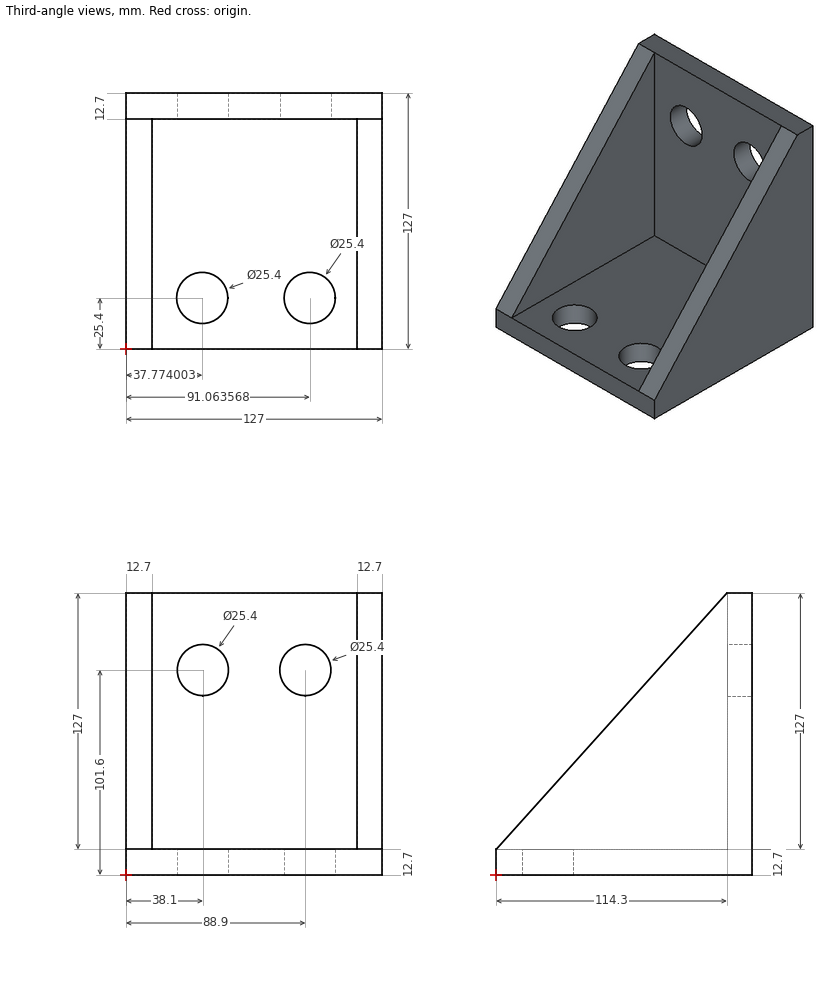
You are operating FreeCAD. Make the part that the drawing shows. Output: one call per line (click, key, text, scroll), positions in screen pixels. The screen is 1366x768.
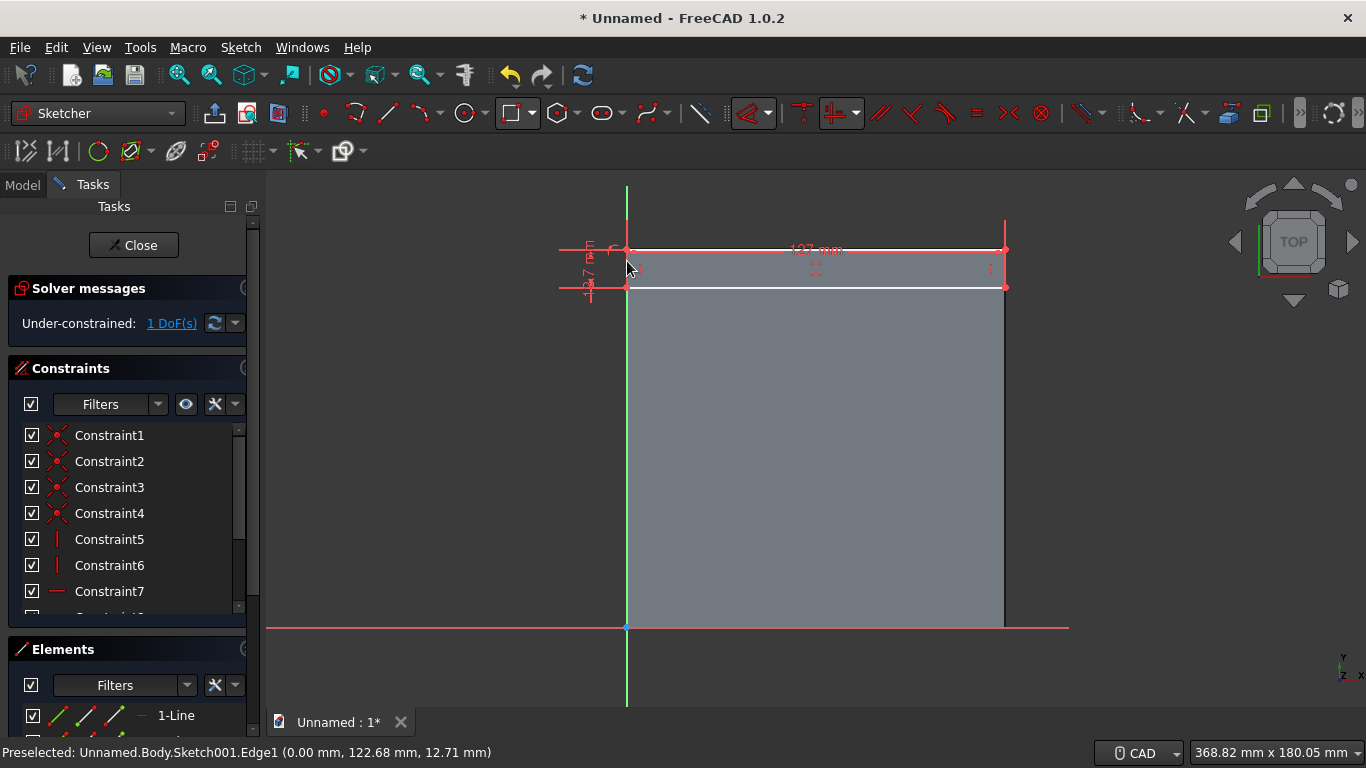
click(627, 250)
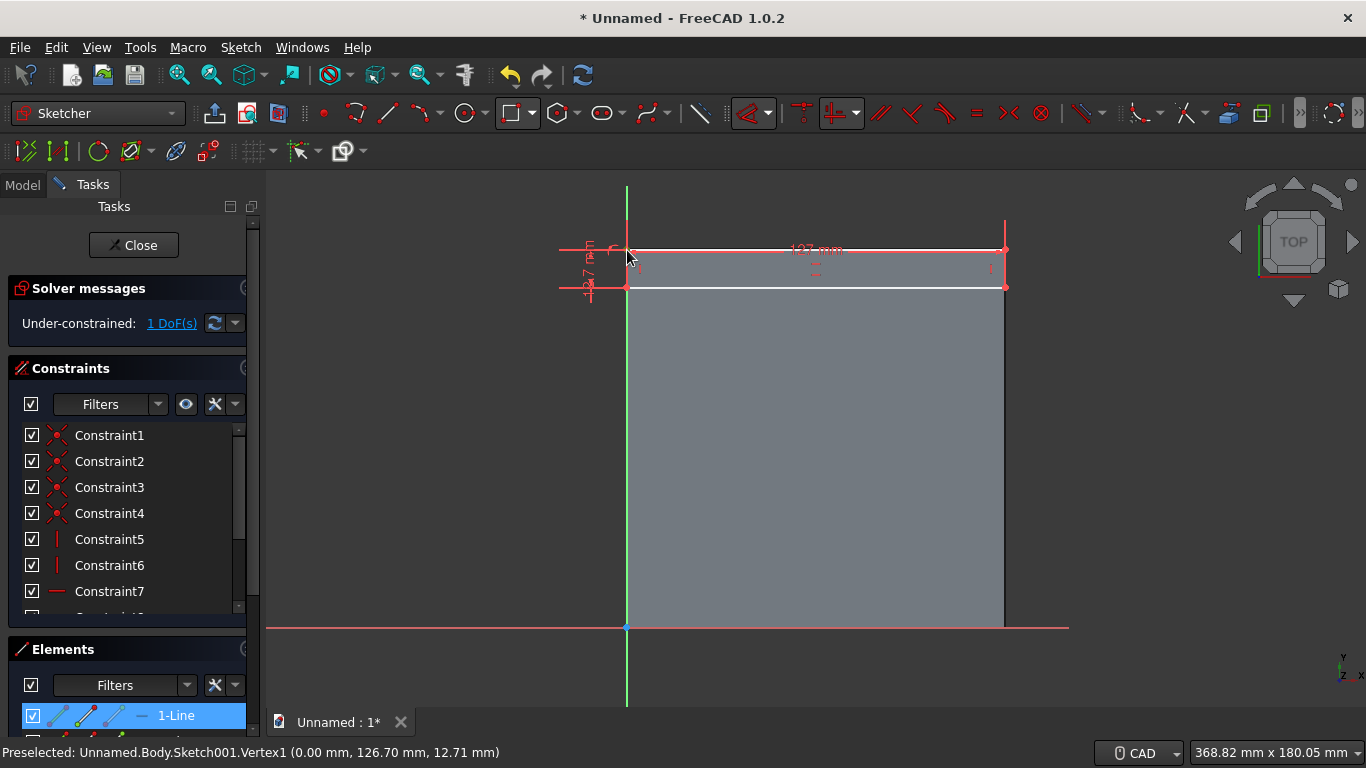
key(i)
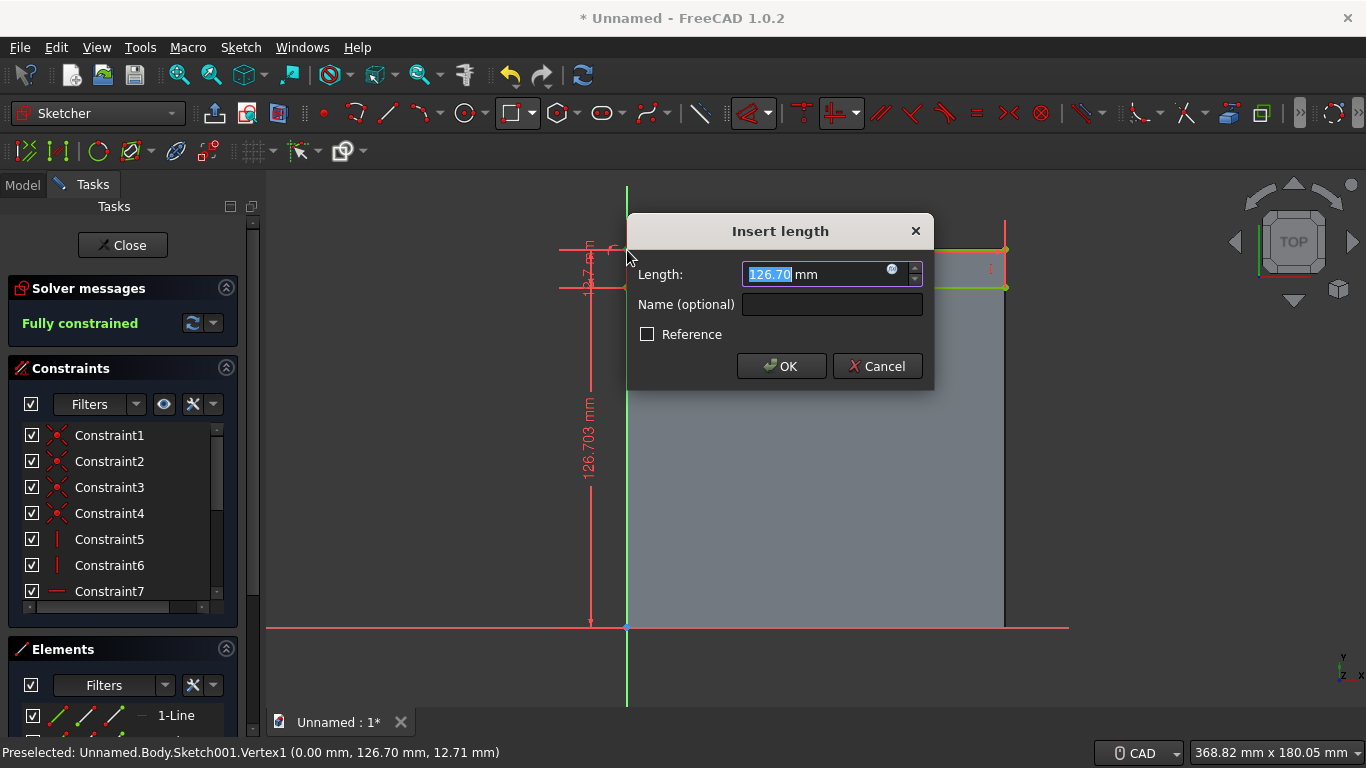
text(127)
key(Return)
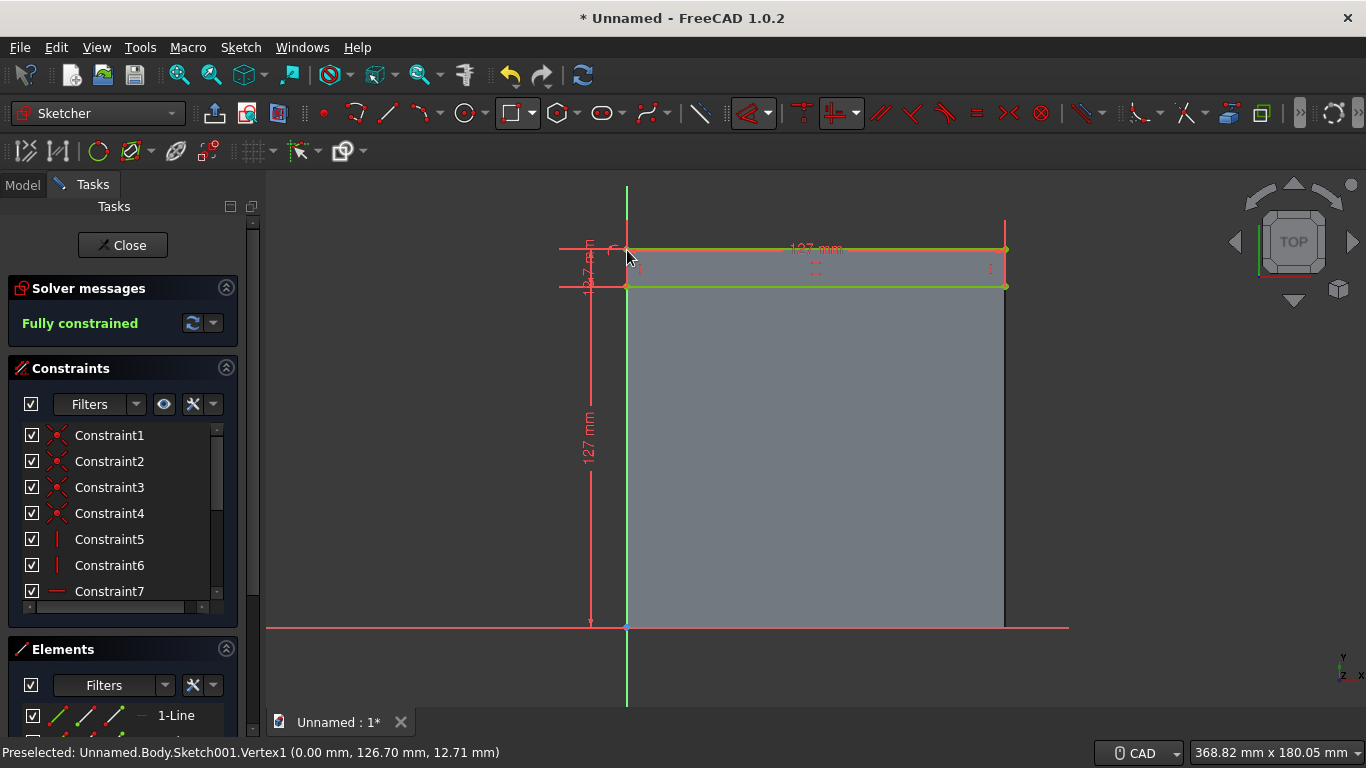
click(123, 245)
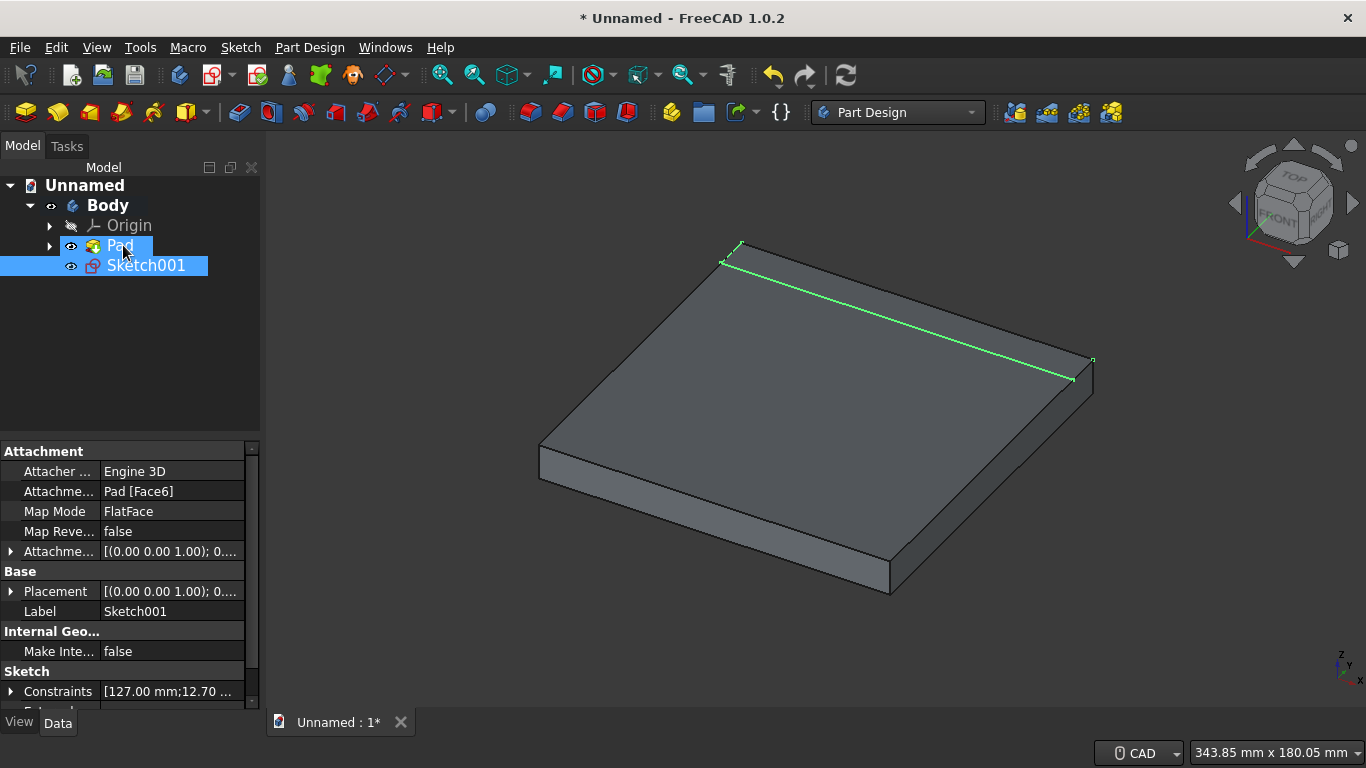
click(26, 112)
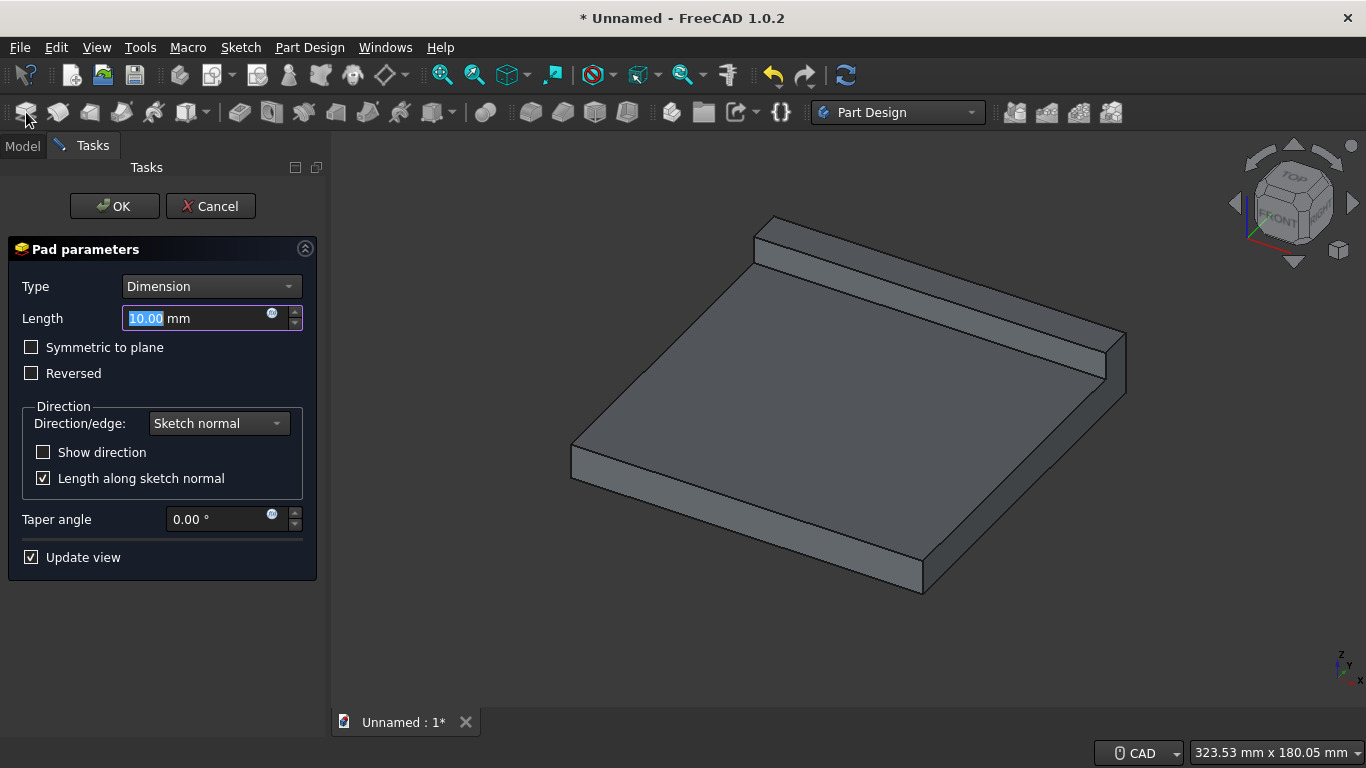
text(127)
key(Tab)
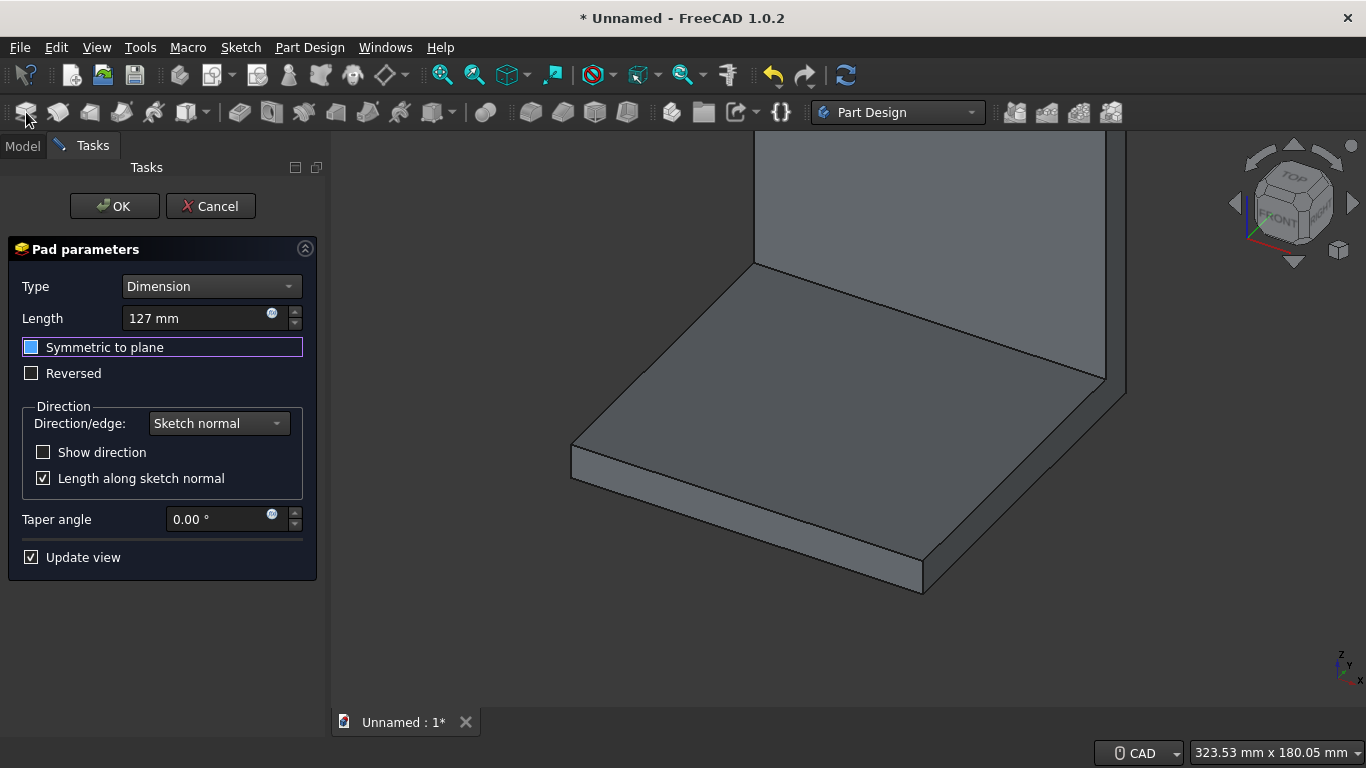
click(115, 206)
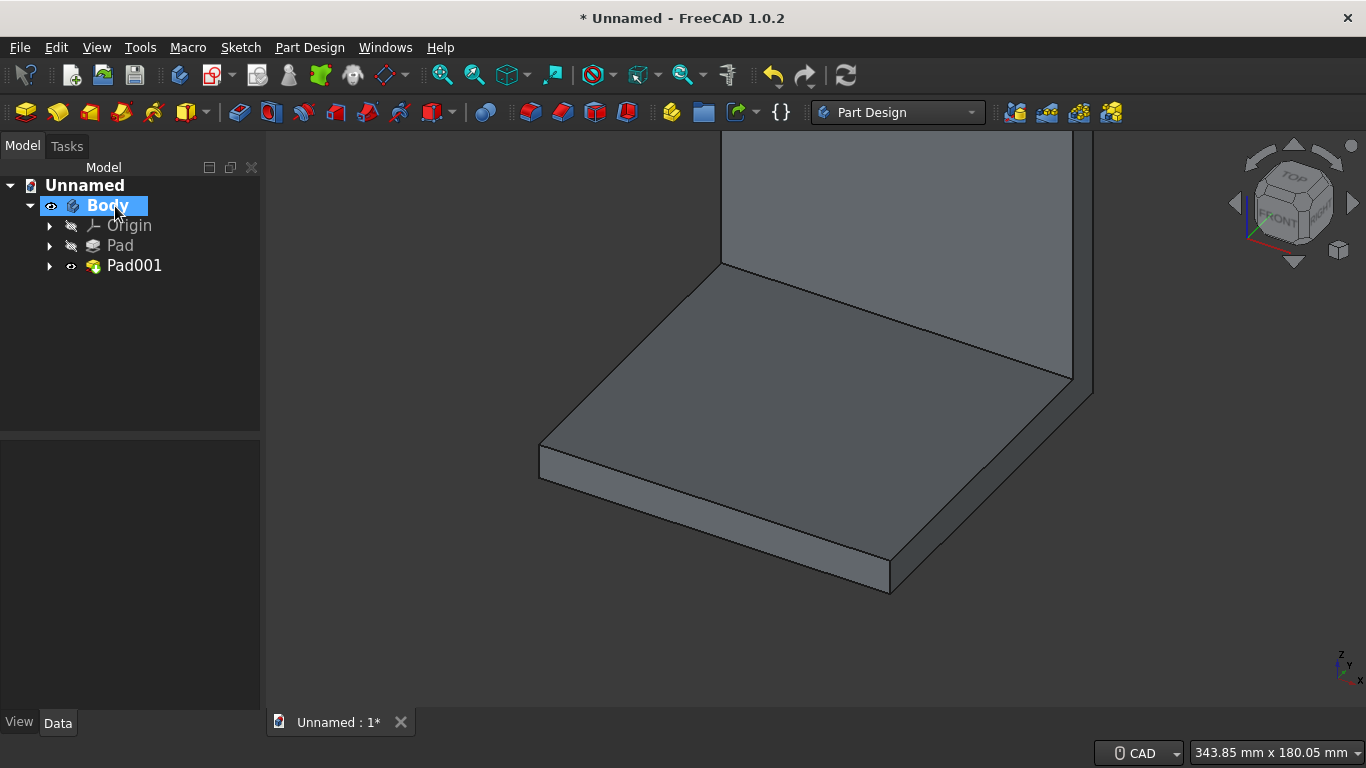
key(v)
key(f)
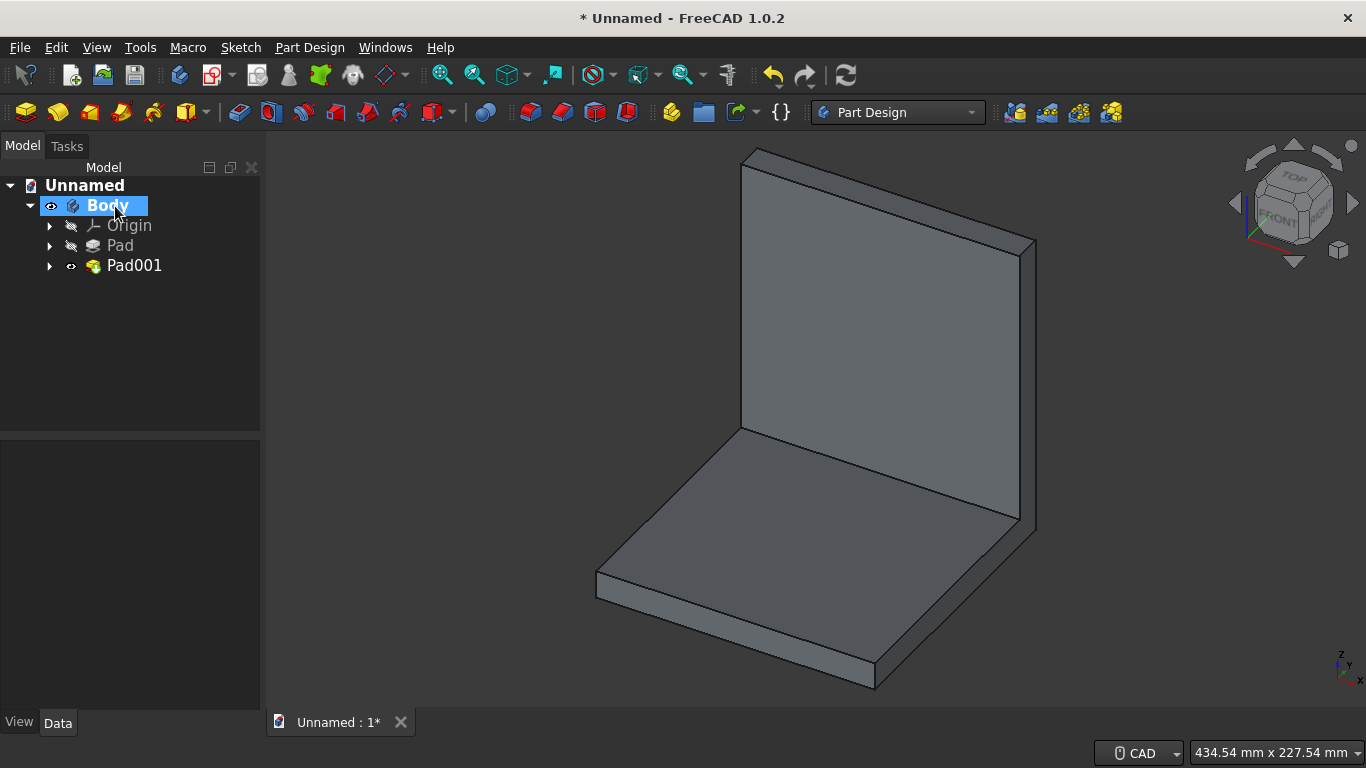
click(212, 76)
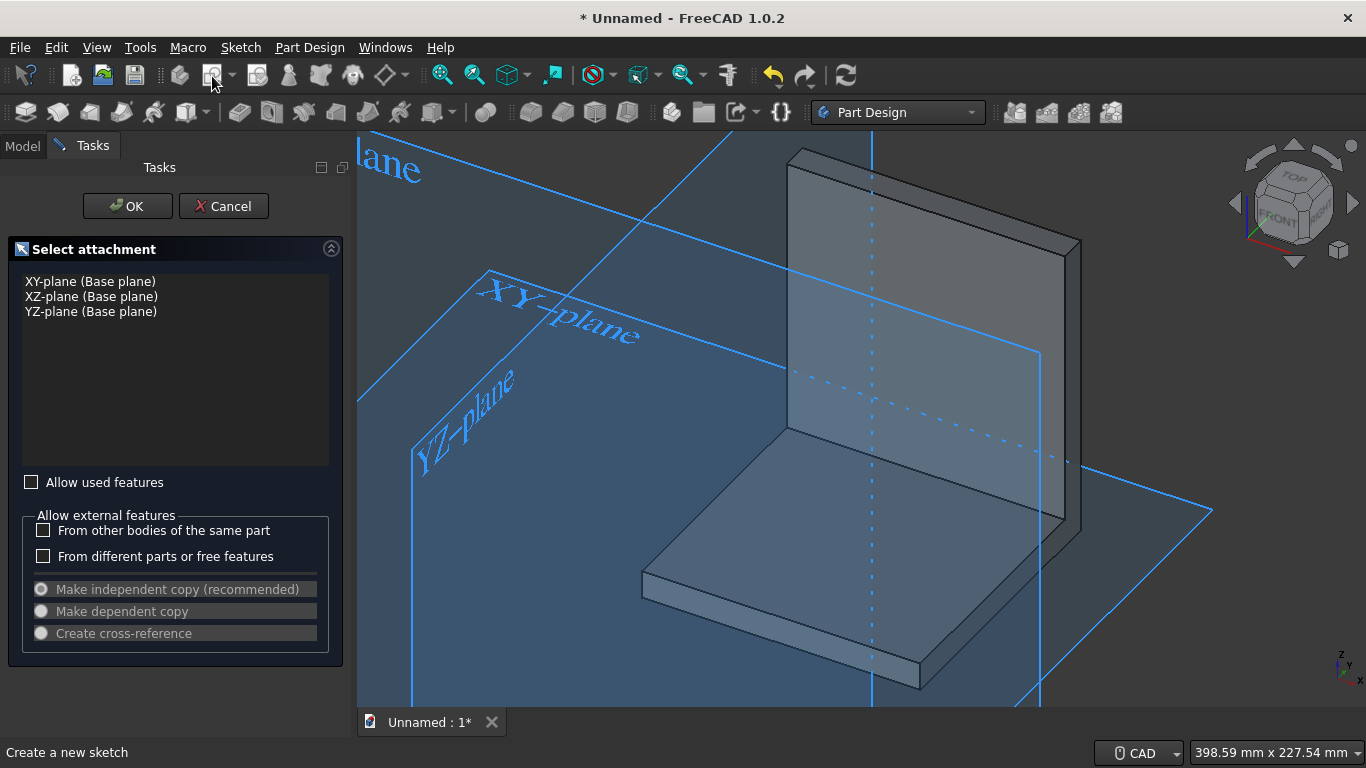
click(82, 312)